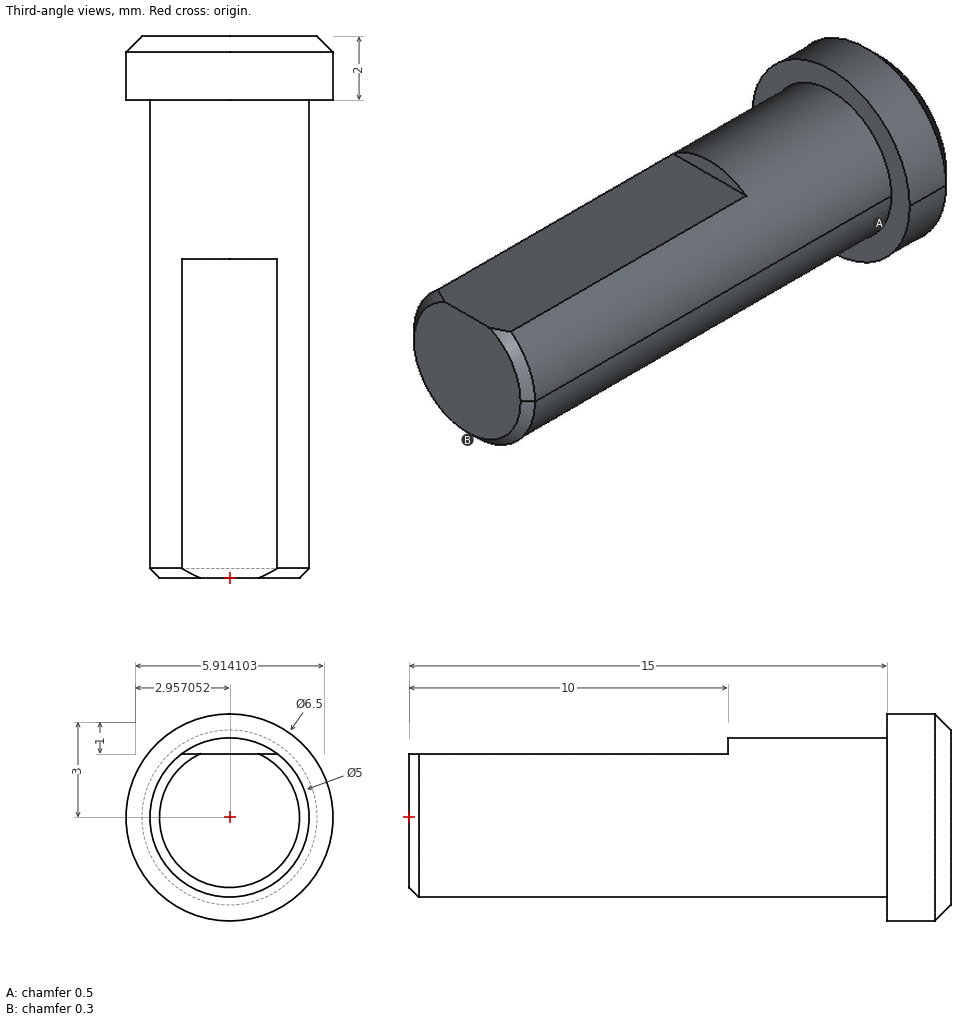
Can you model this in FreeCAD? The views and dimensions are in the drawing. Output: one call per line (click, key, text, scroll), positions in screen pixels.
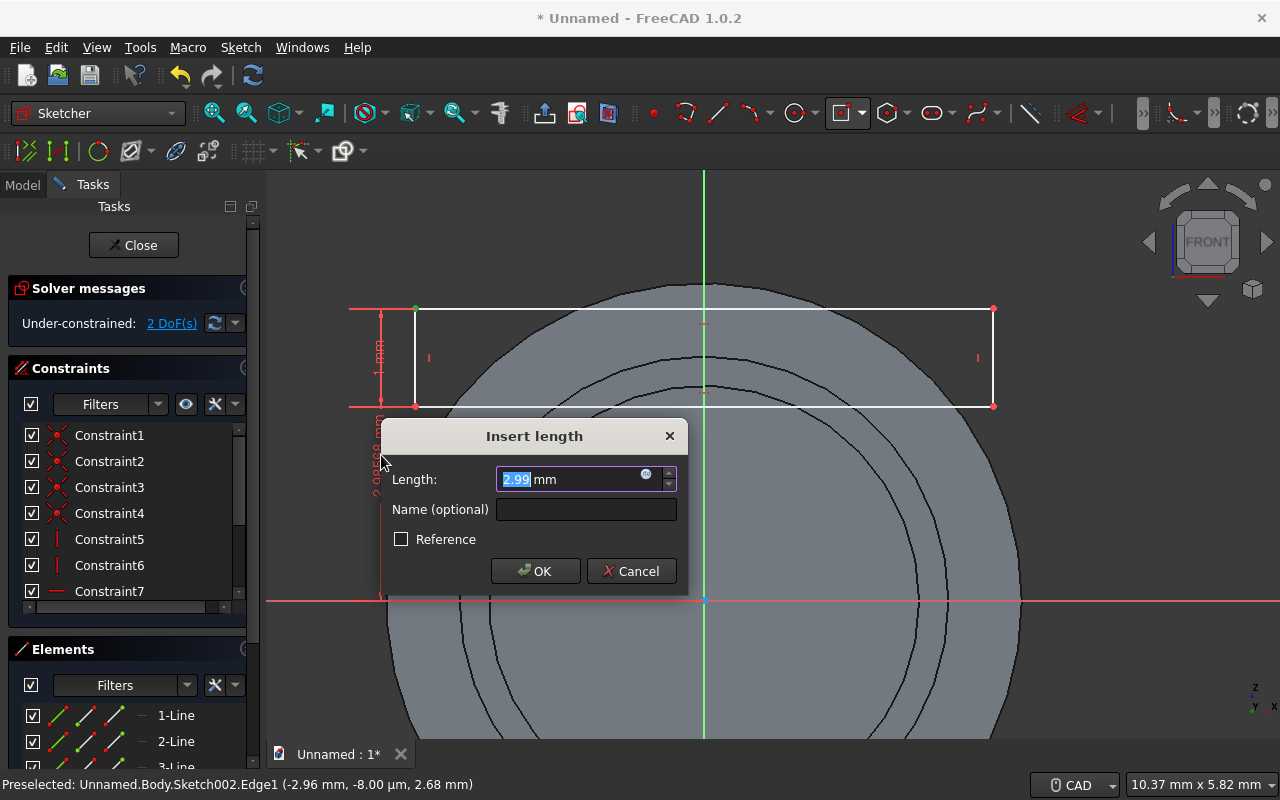
text(3)
key(Return)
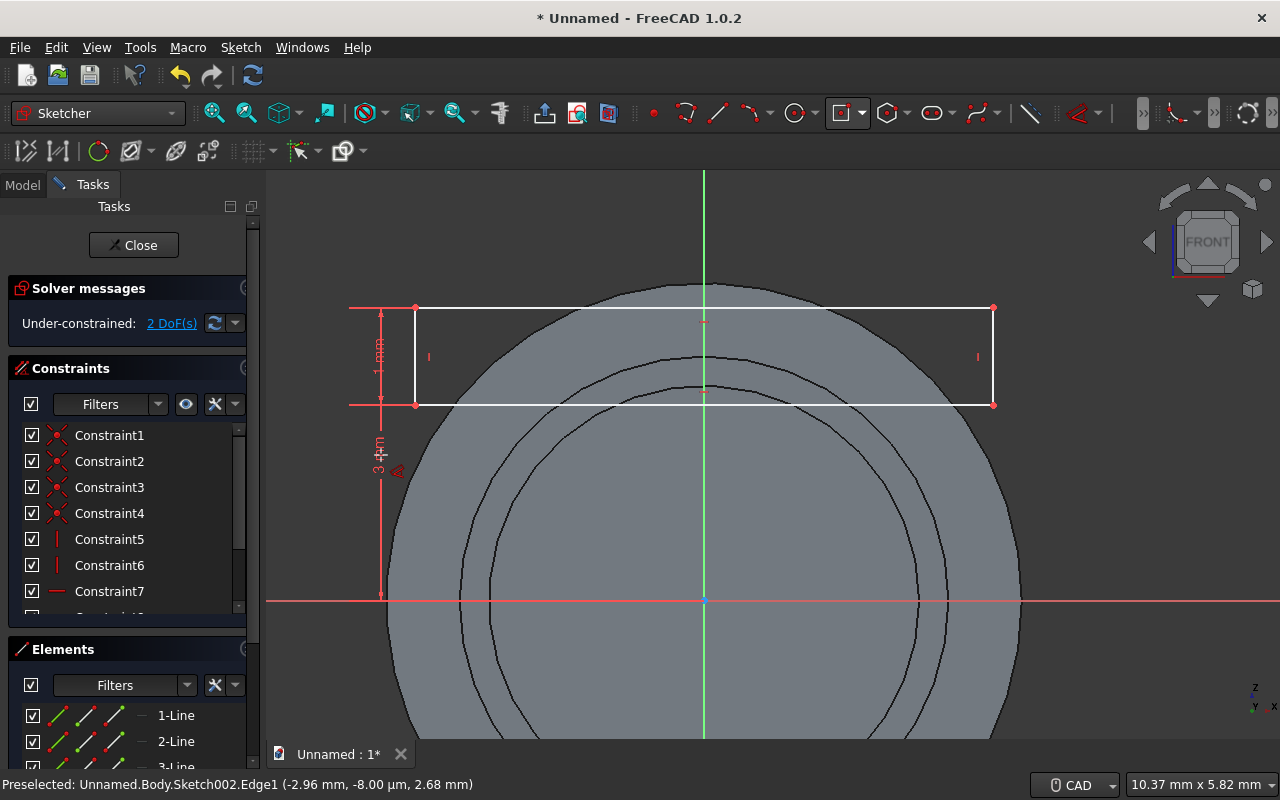
click(588, 405)
click(571, 371)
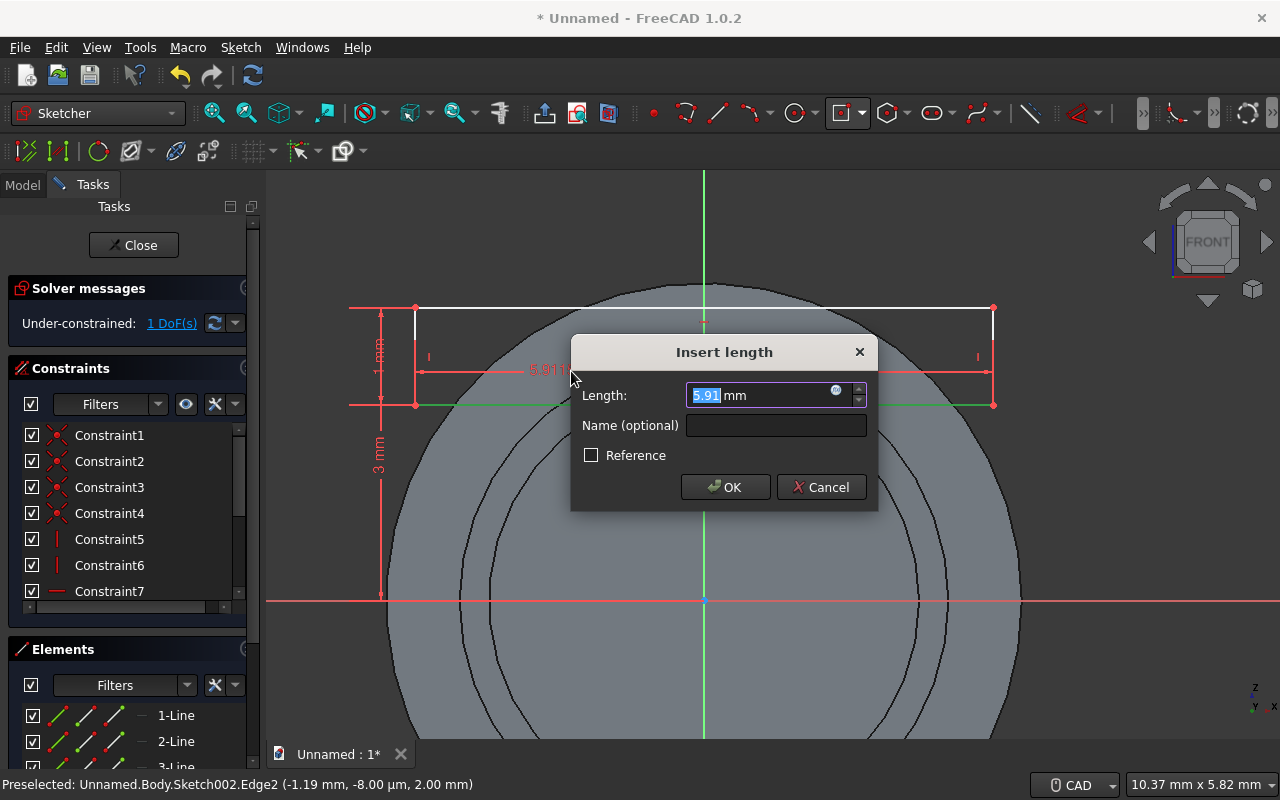
text(5.914103)
key(Return)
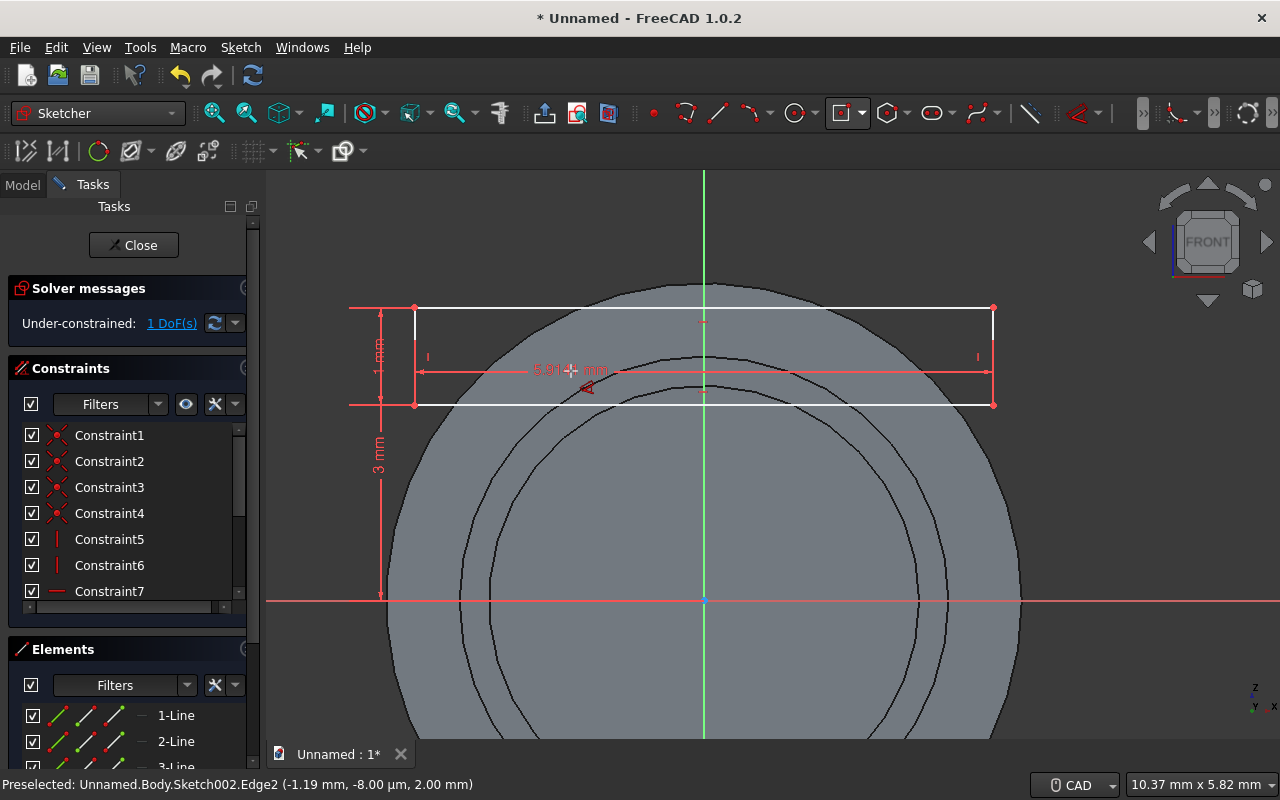
click(415, 308)
click(559, 635)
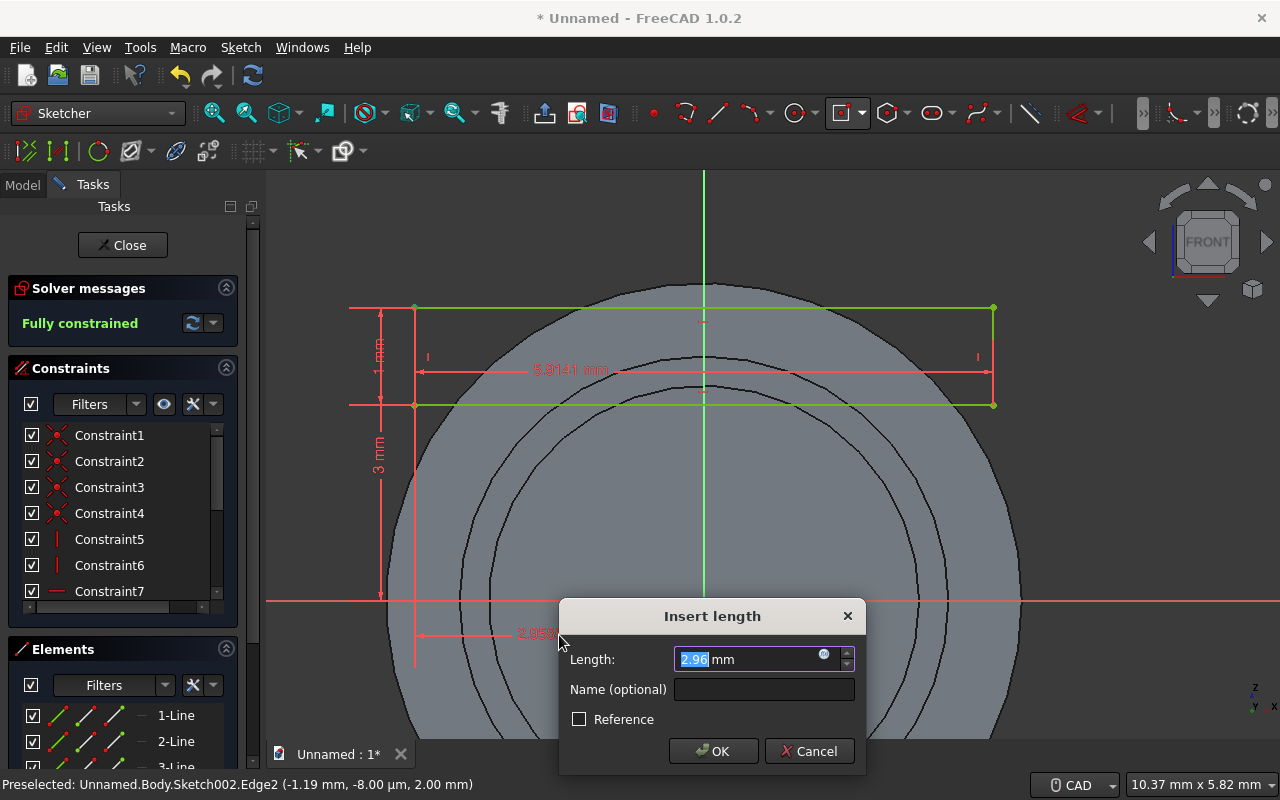
text(2.957052)
key(Return)
key(Escape)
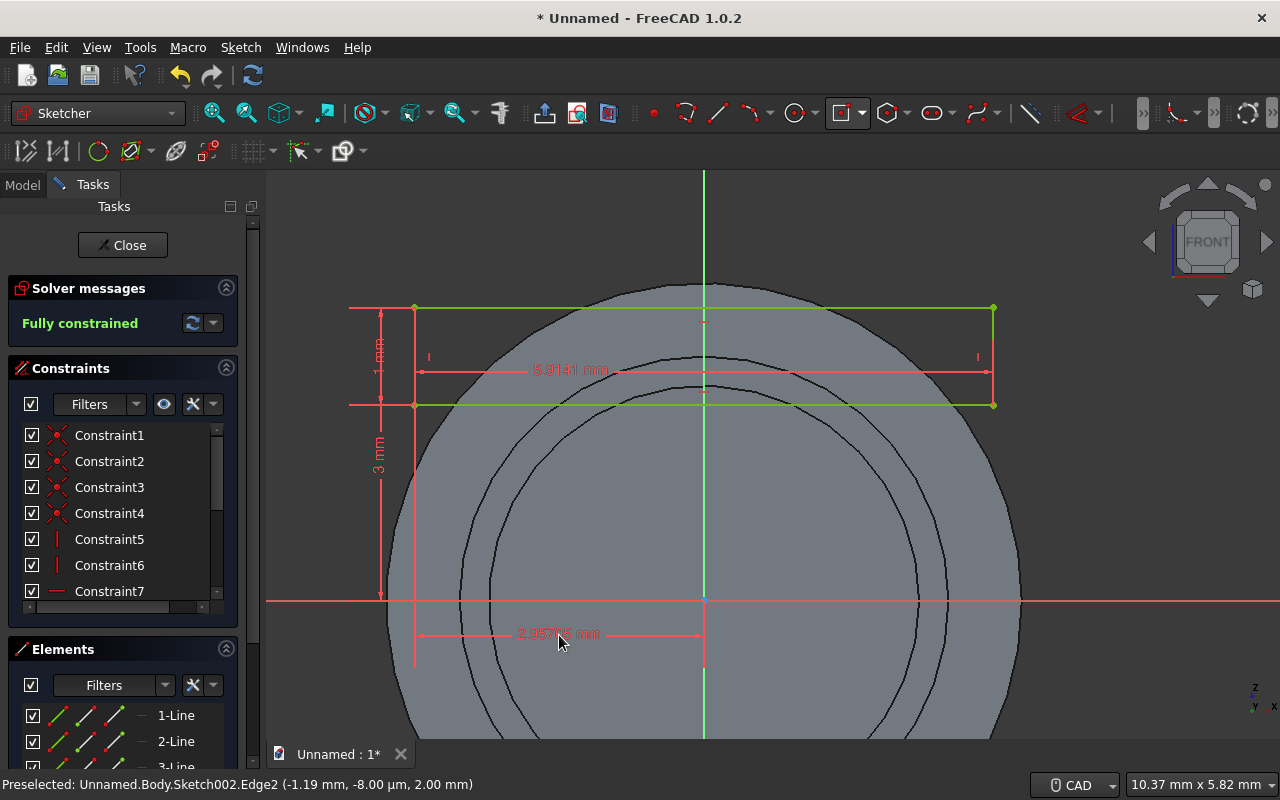
click(123, 245)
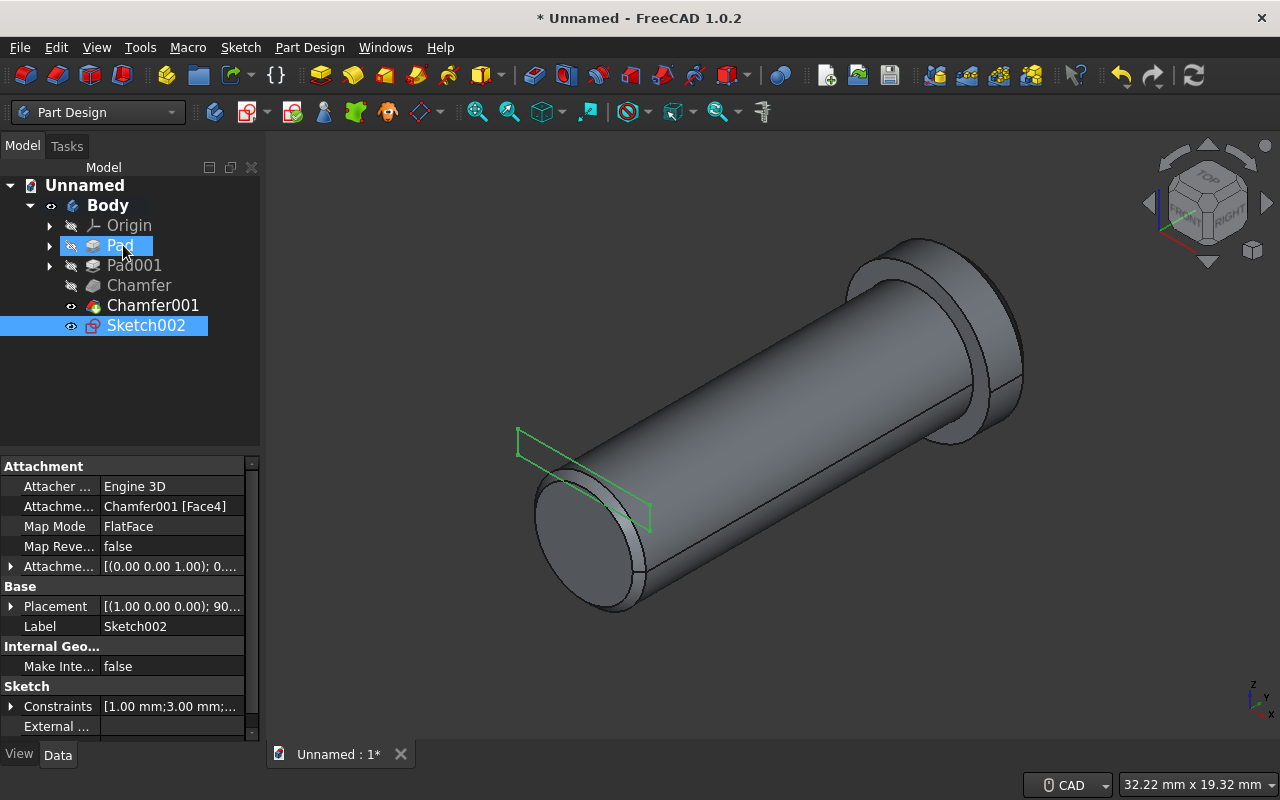
click(536, 76)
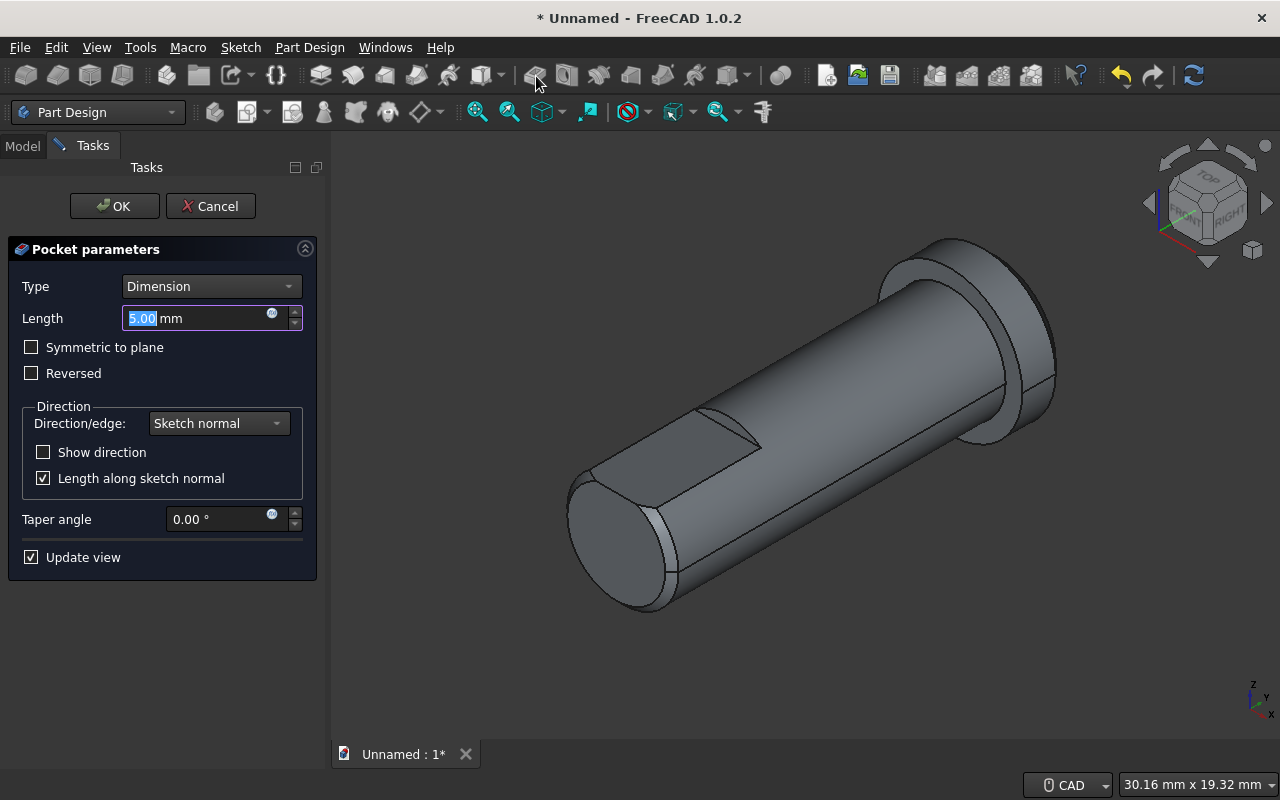
text(10)
key(Tab)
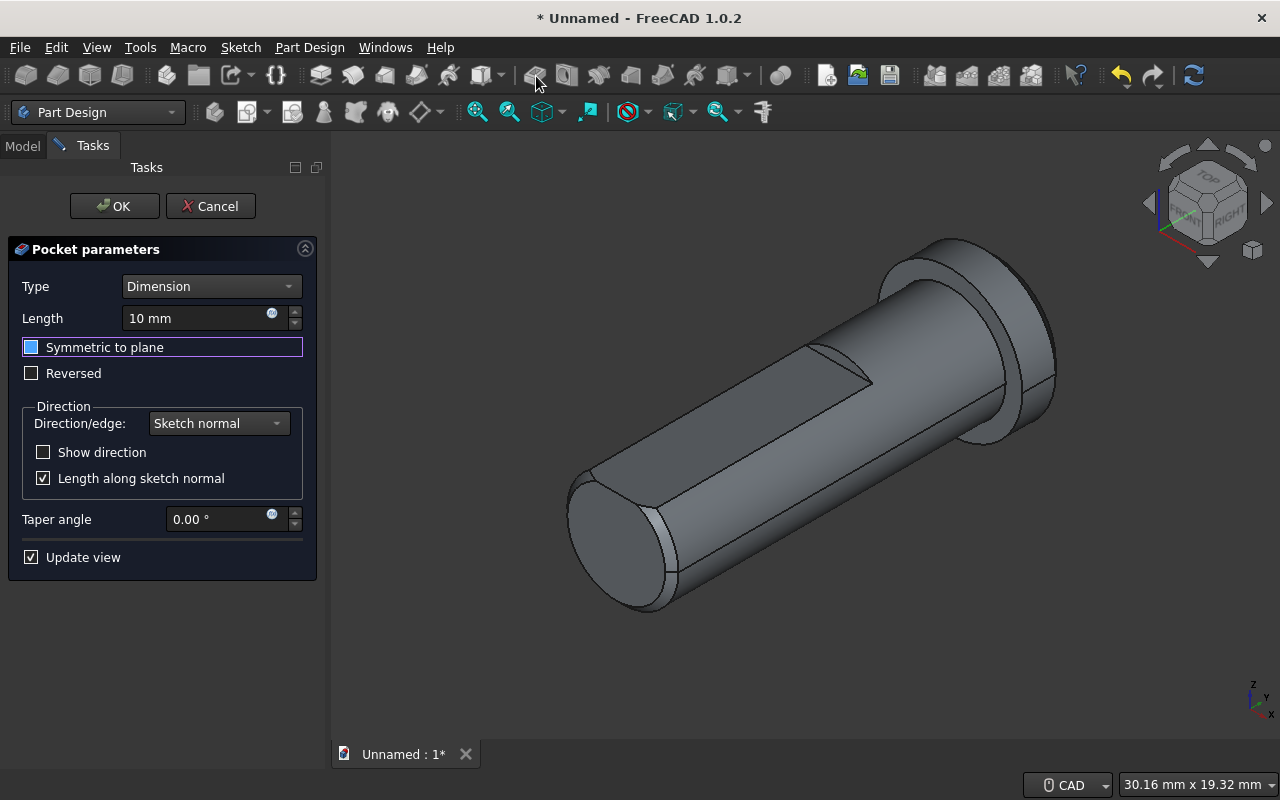
click(115, 206)